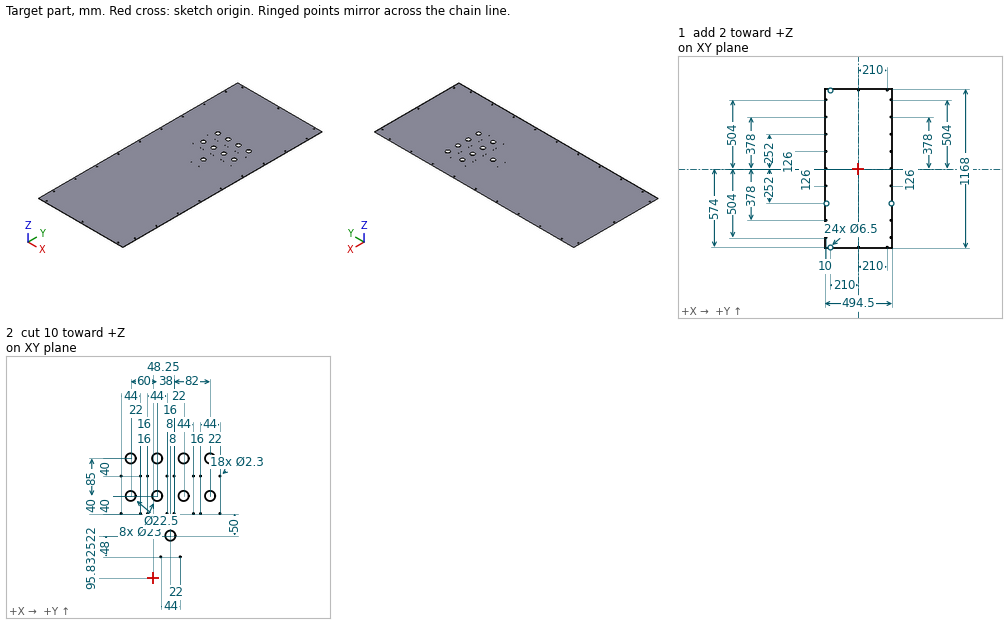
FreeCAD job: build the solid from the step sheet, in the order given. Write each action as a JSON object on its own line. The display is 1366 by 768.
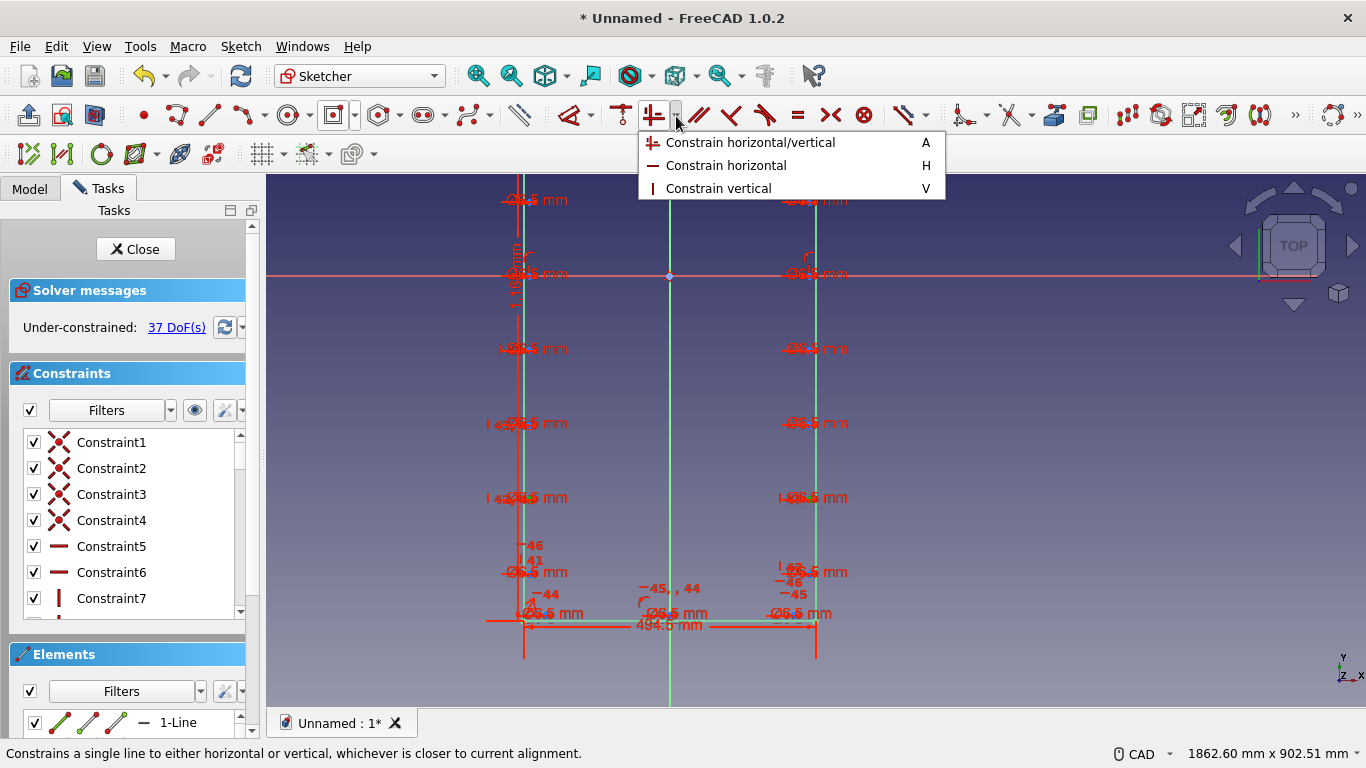
{"action": "left_click", "coordinate": [792, 166]}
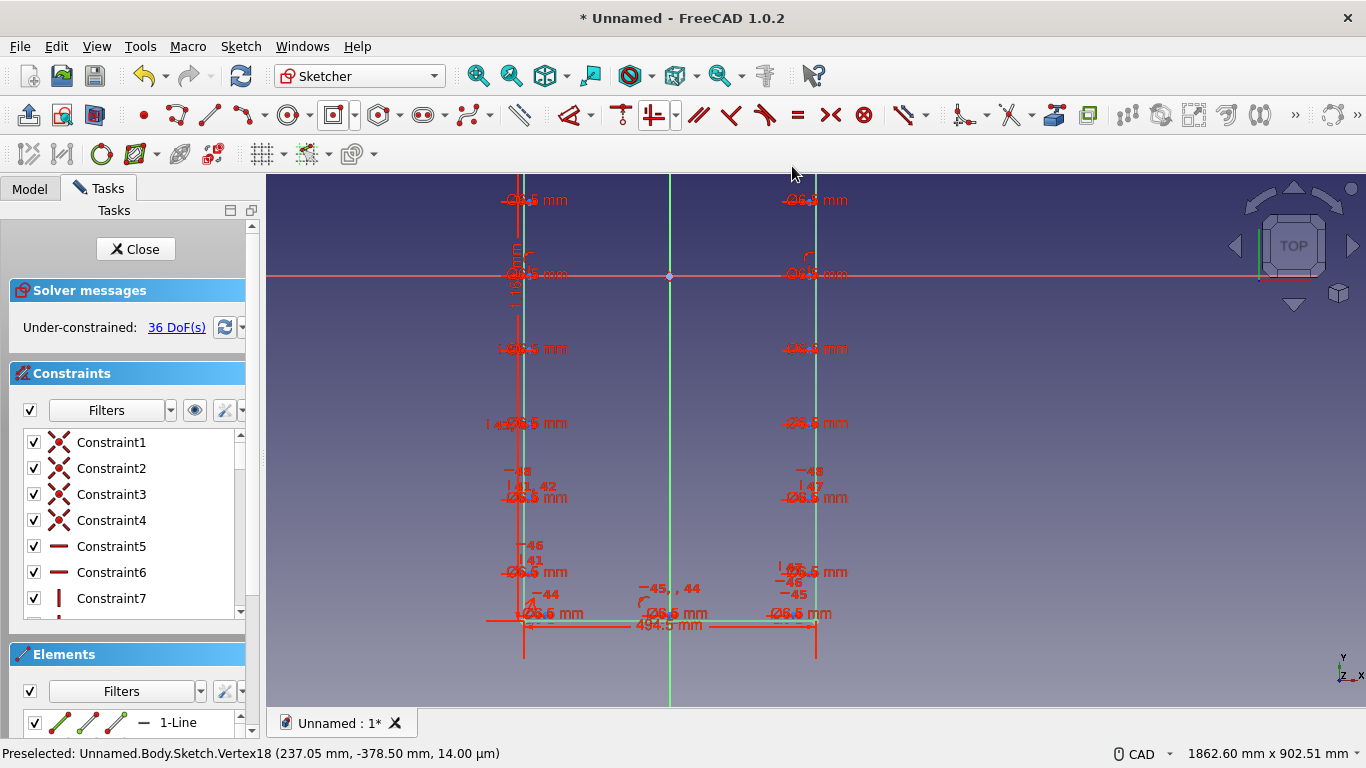
{"action": "left_click", "coordinate": [810, 500]}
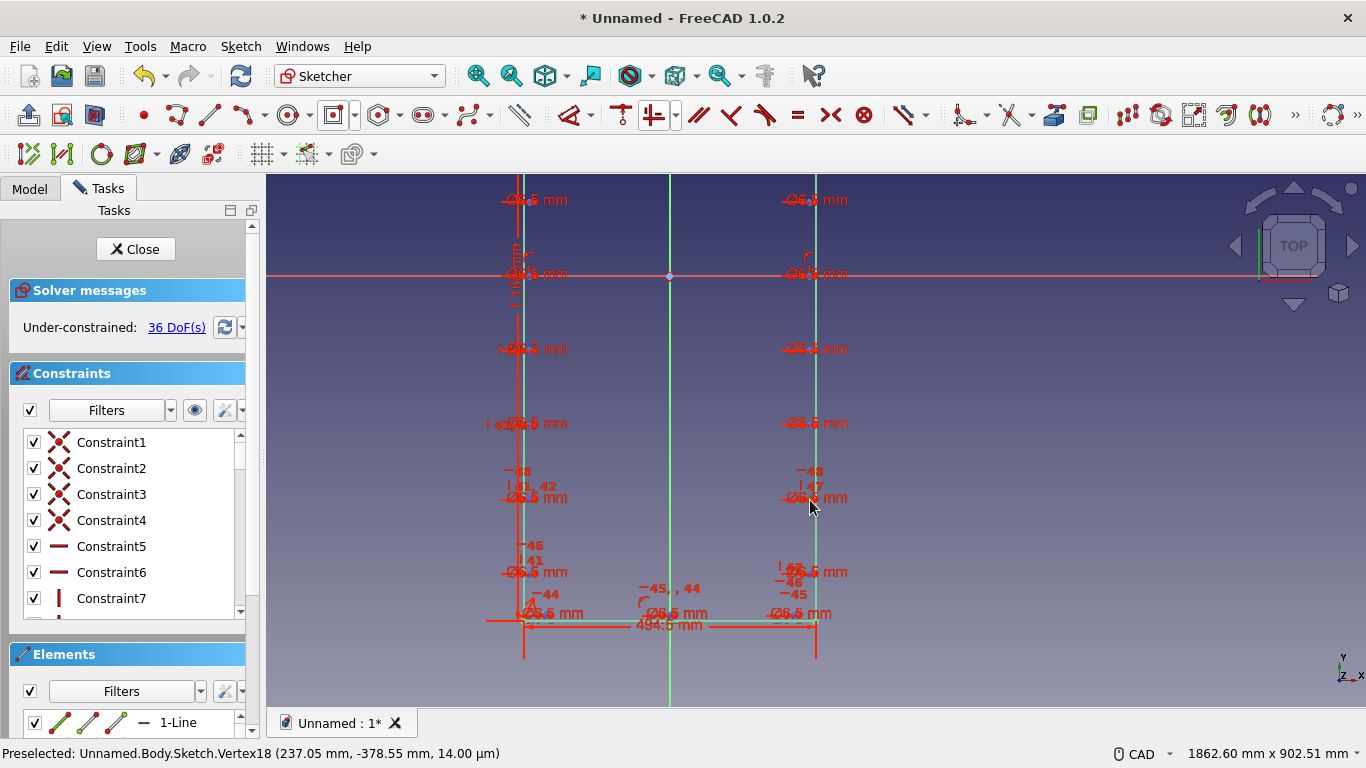
{"action": "left_click", "coordinate": [810, 425]}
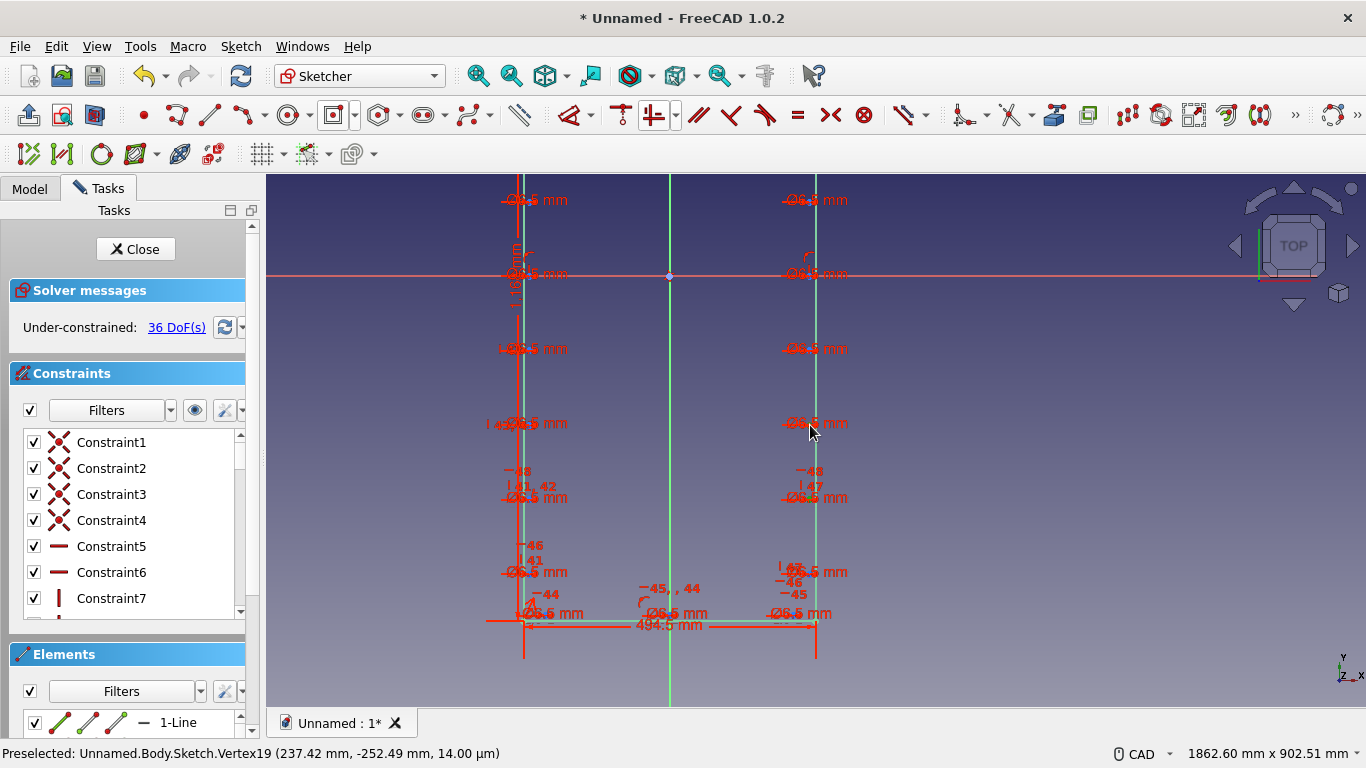
{"action": "left_click", "coordinate": [676, 116]}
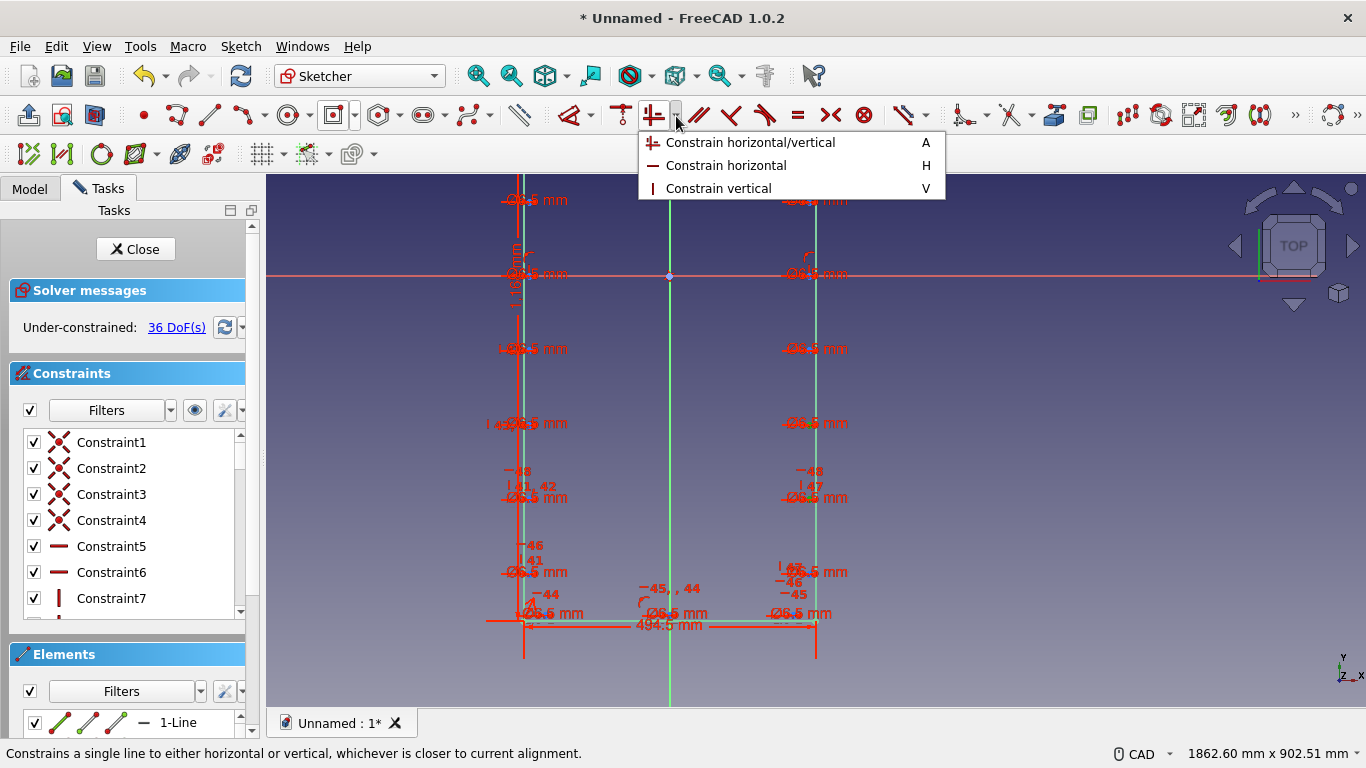
{"action": "left_click", "coordinate": [792, 188]}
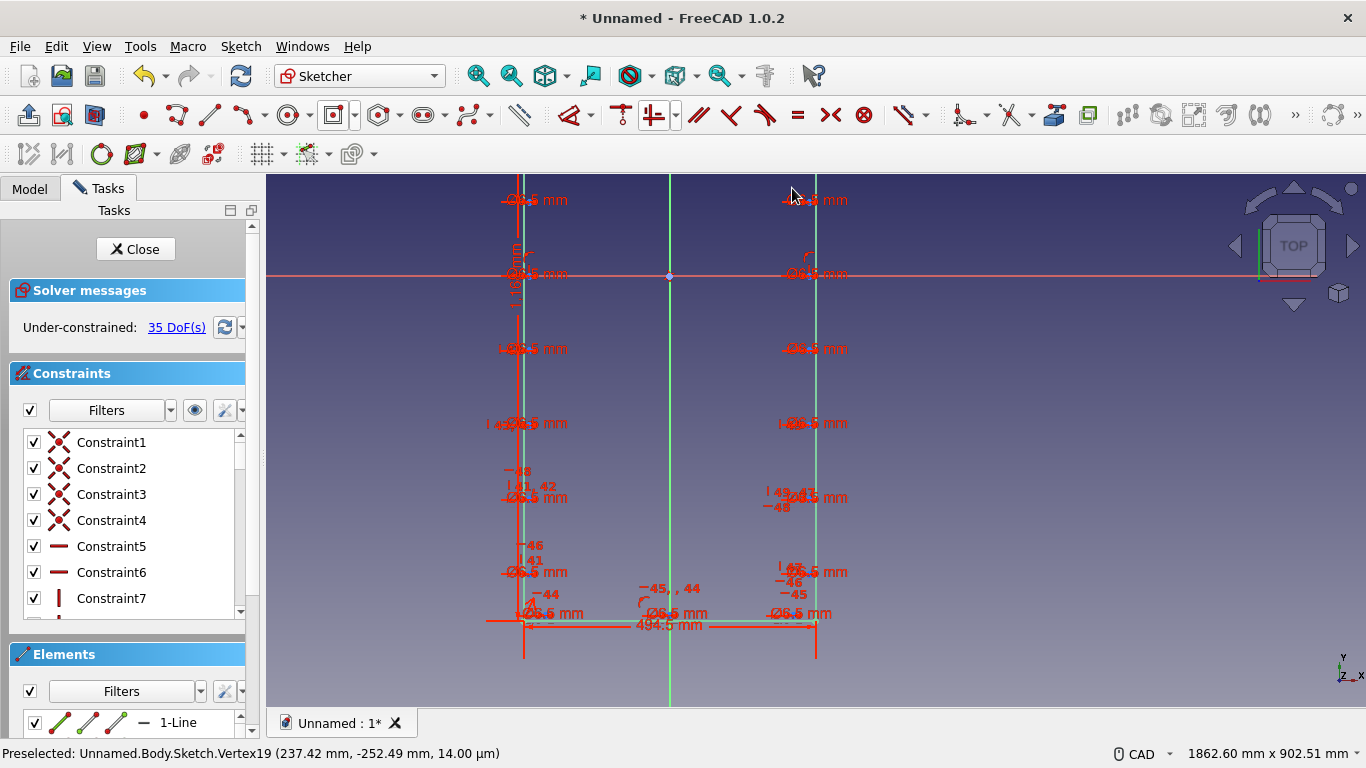
{"action": "left_click", "coordinate": [810, 425]}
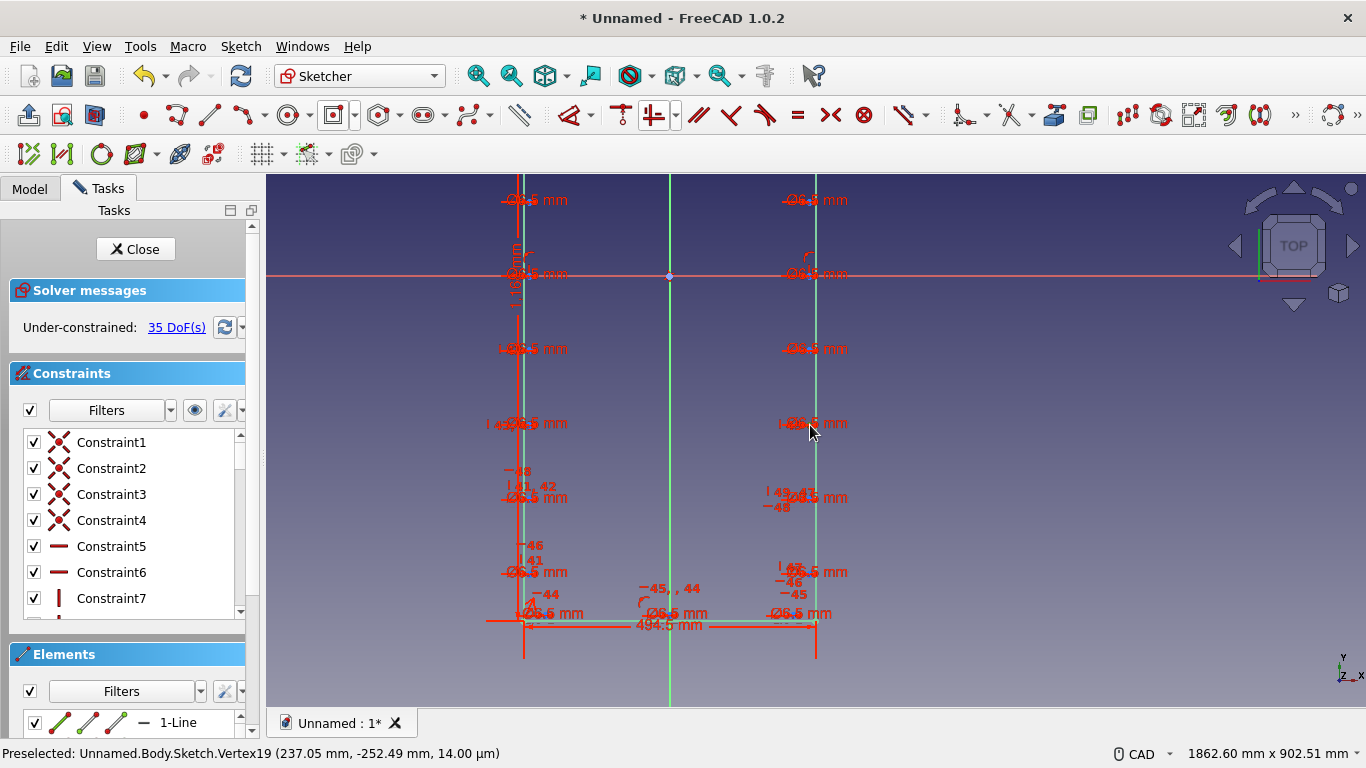
{"action": "left_click", "coordinate": [810, 351]}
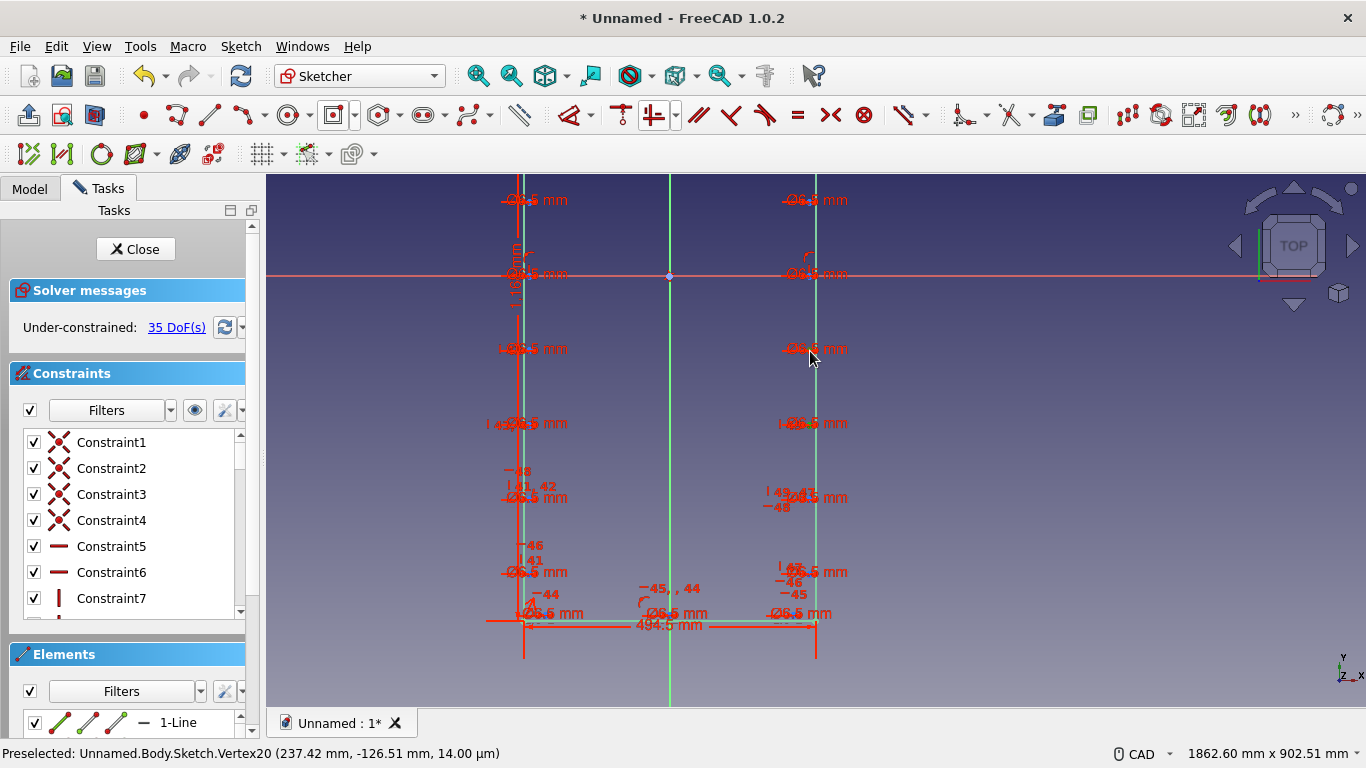
{"action": "left_click", "coordinate": [676, 116]}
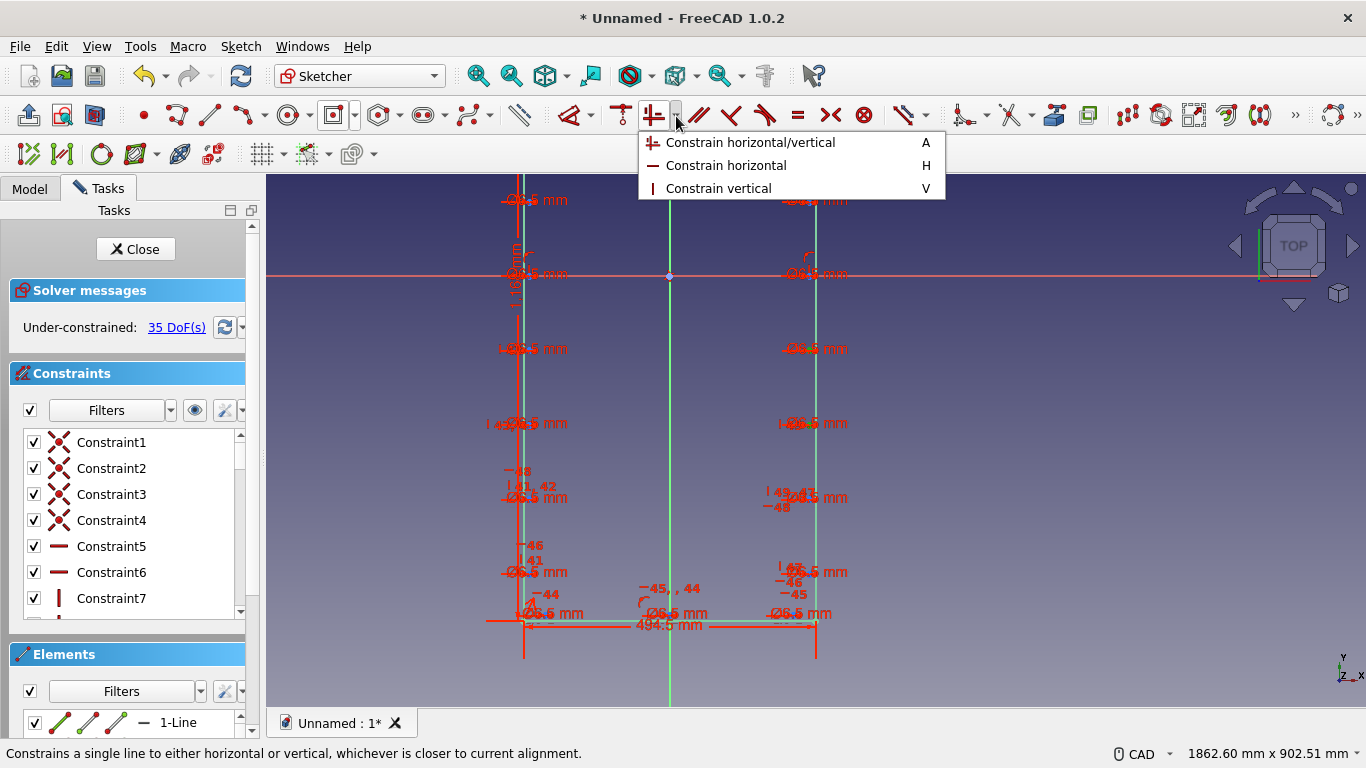
{"action": "left_click", "coordinate": [792, 188]}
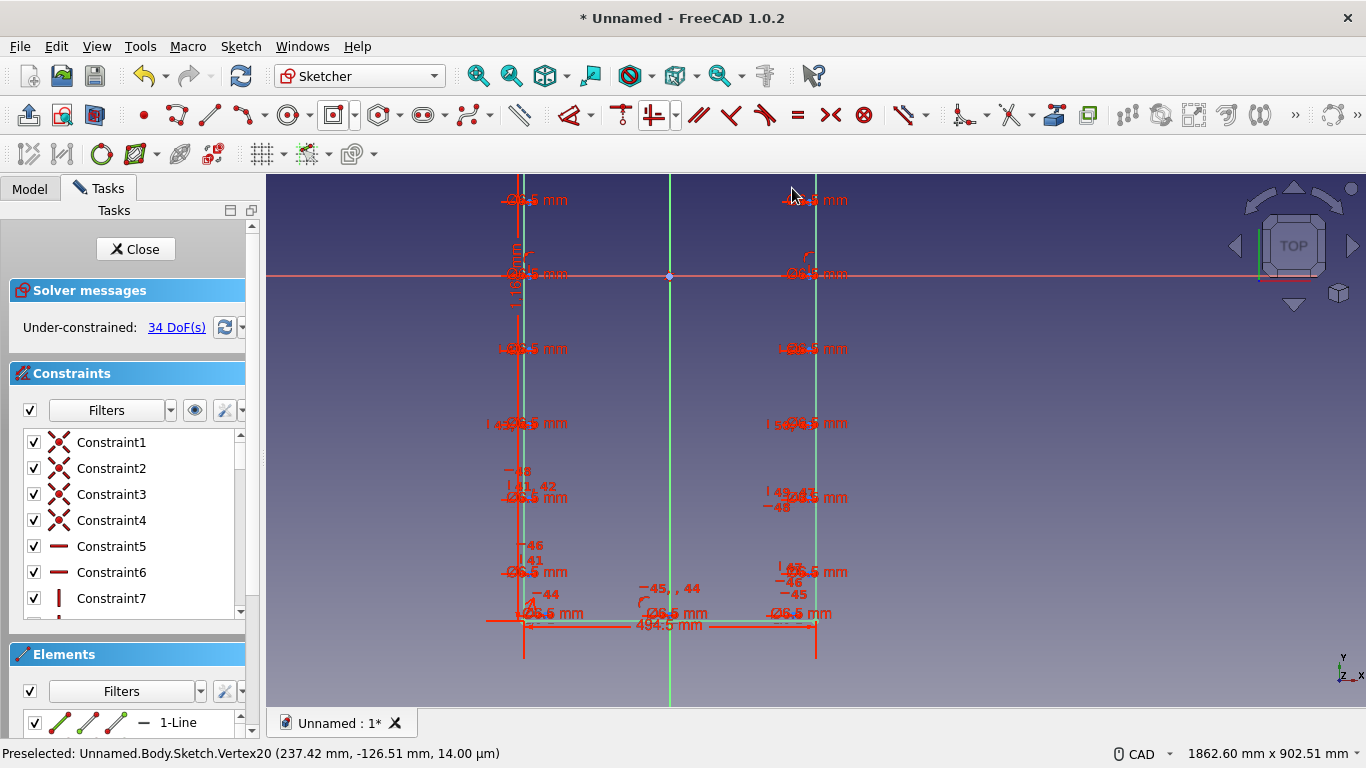
{"action": "left_click", "coordinate": [530, 351]}